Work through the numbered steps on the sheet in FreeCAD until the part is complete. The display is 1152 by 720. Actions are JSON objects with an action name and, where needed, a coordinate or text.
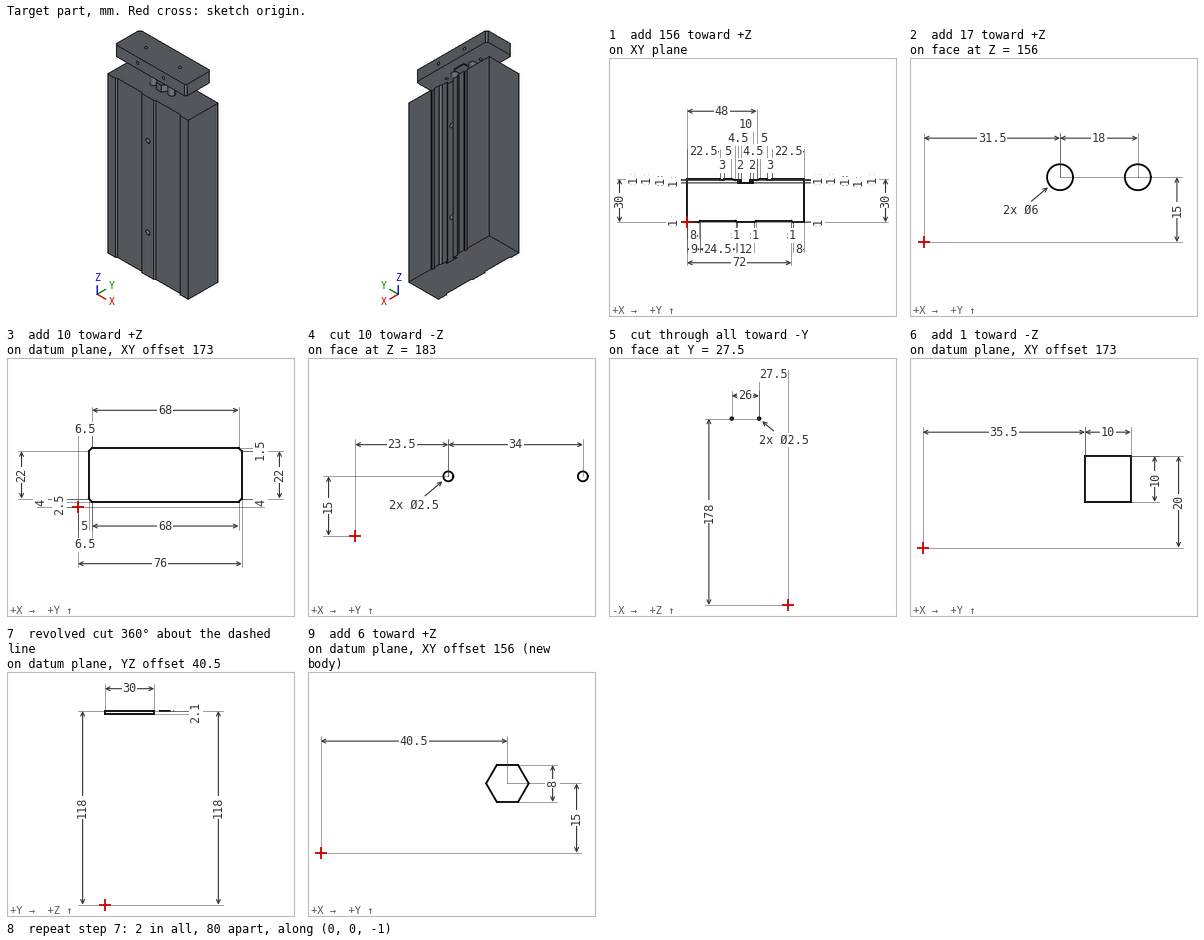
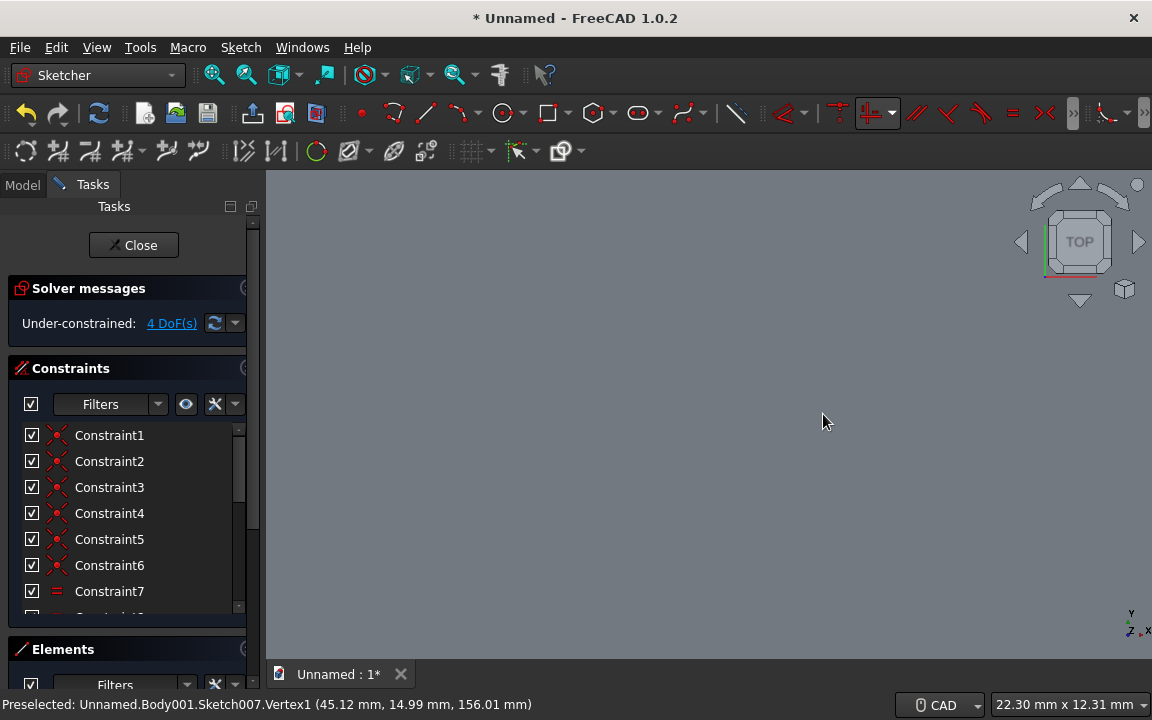
{"action": "left_click", "coordinate": [676, 256]}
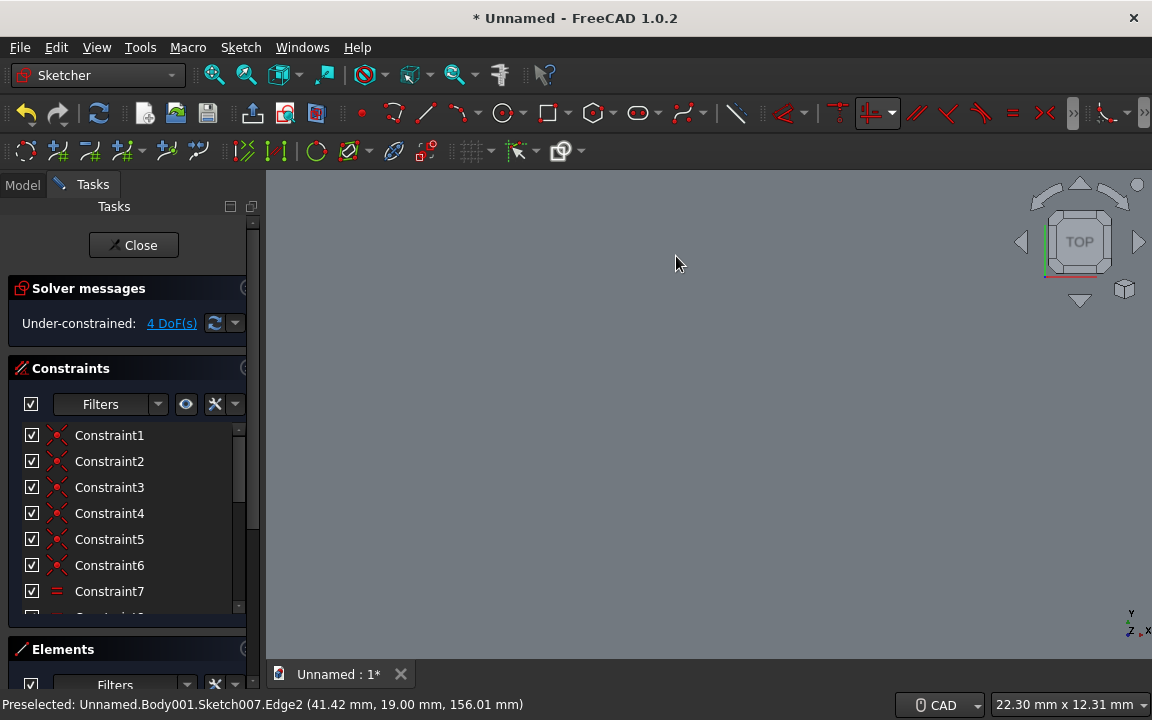
{"action": "key", "text": "h"}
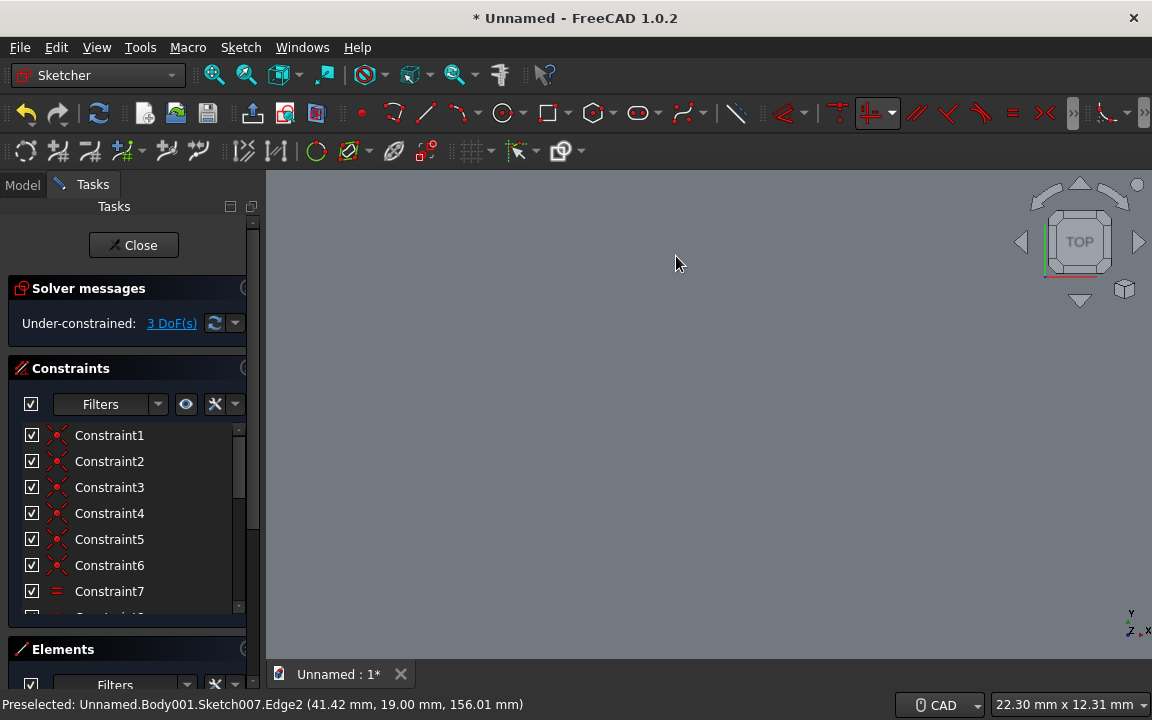
{"action": "left_click", "coordinate": [784, 114]}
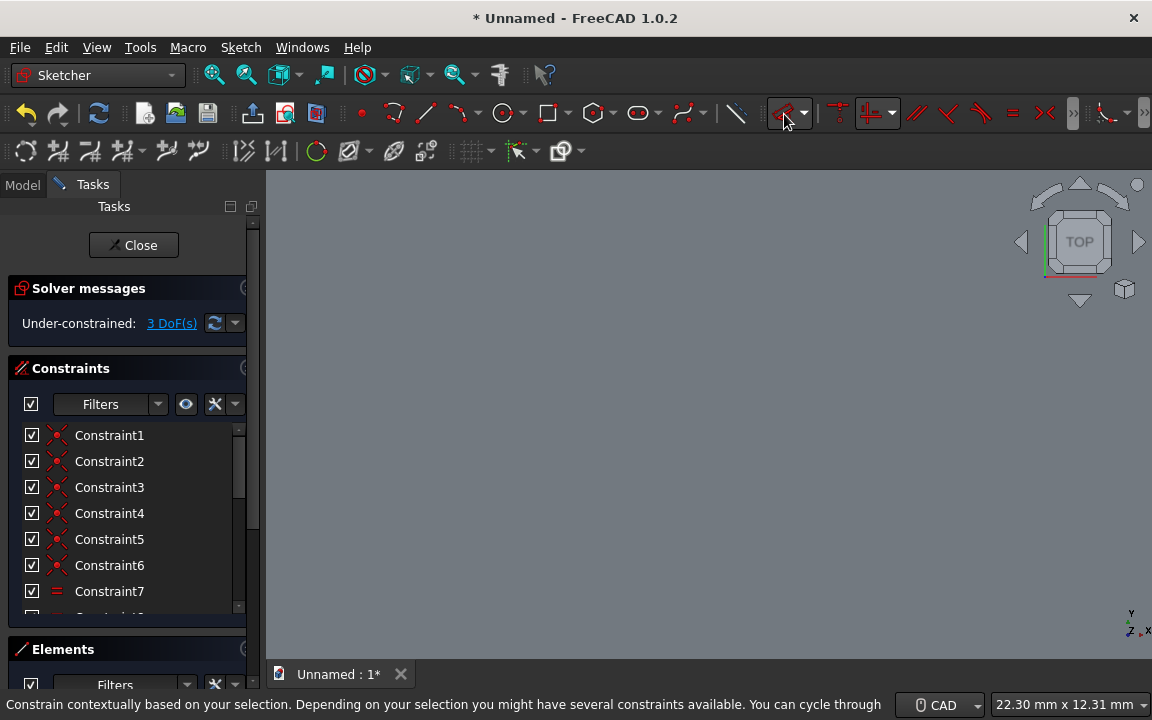
{"action": "left_click", "coordinate": [547, 574]}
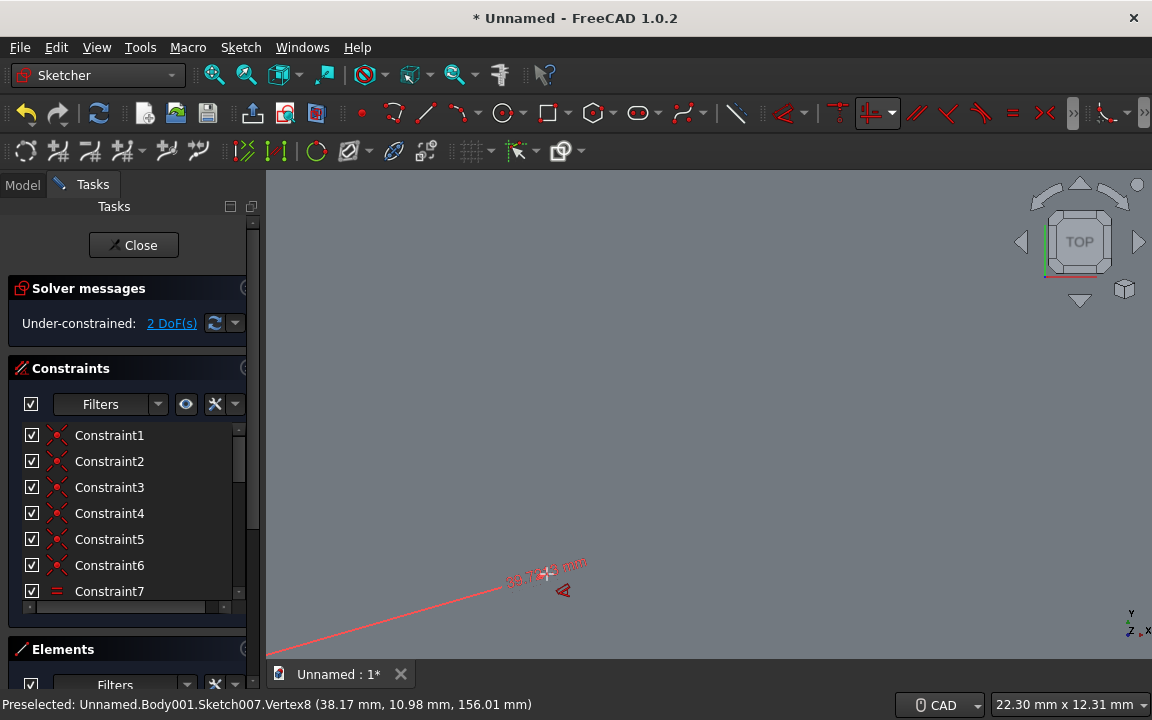
{"action": "left_click", "coordinate": [731, 256]}
{"action": "left_click", "coordinate": [513, 415]}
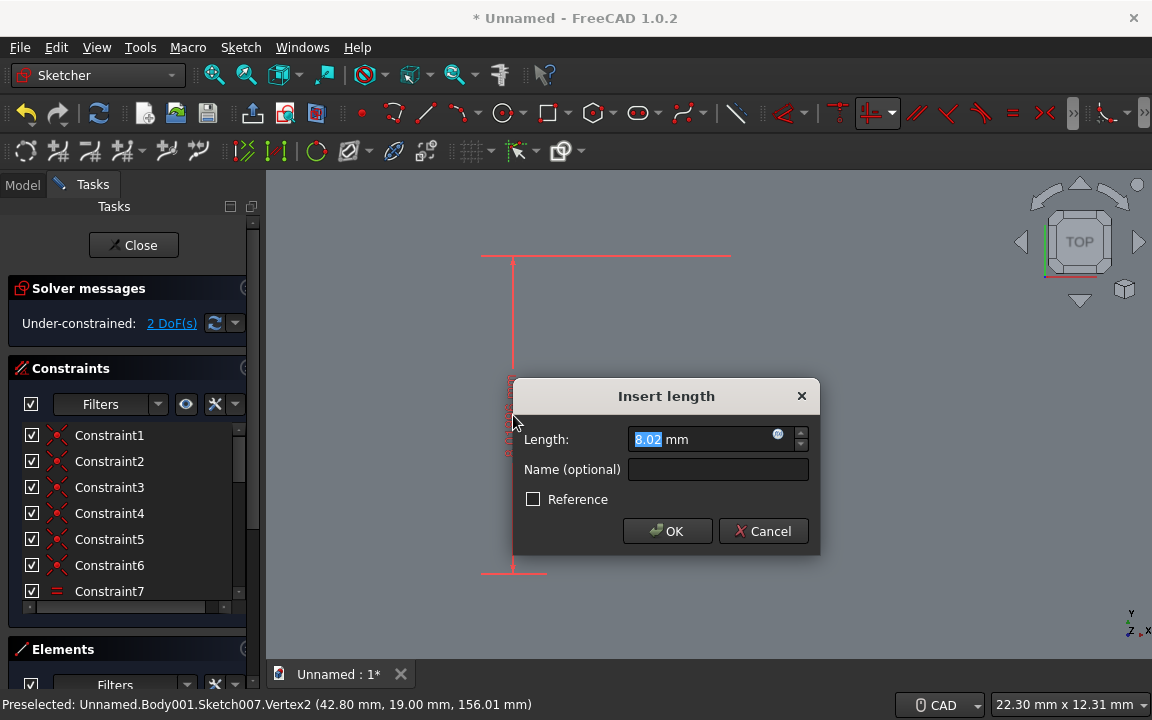
{"action": "type", "text": "8"}
{"action": "key", "text": "Return"}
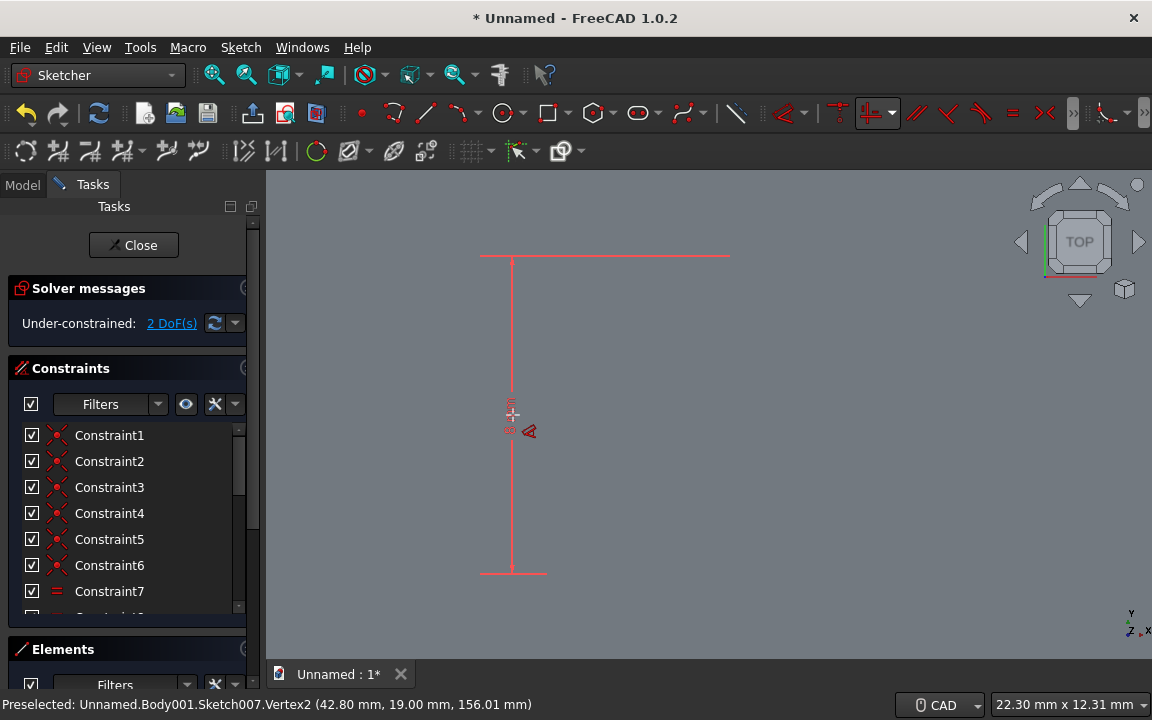
{"action": "left_click", "coordinate": [639, 415]}
{"action": "left_click", "coordinate": [673, 523]}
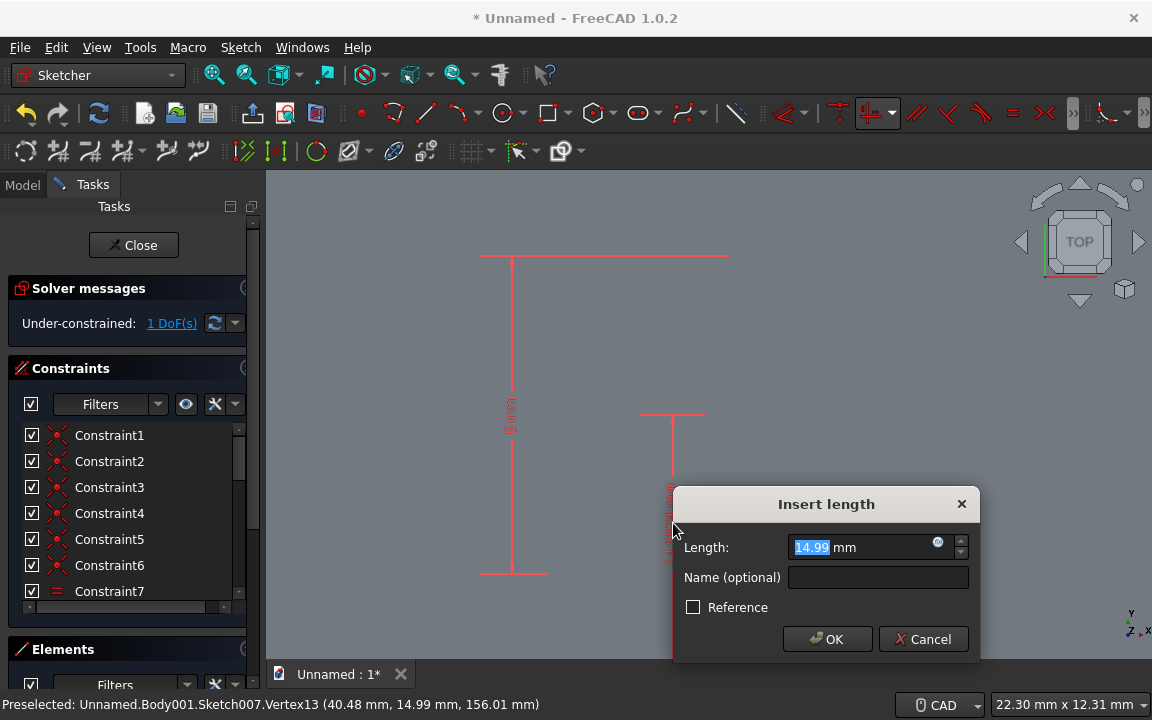
{"action": "type", "text": "15"}
{"action": "key", "text": "Return"}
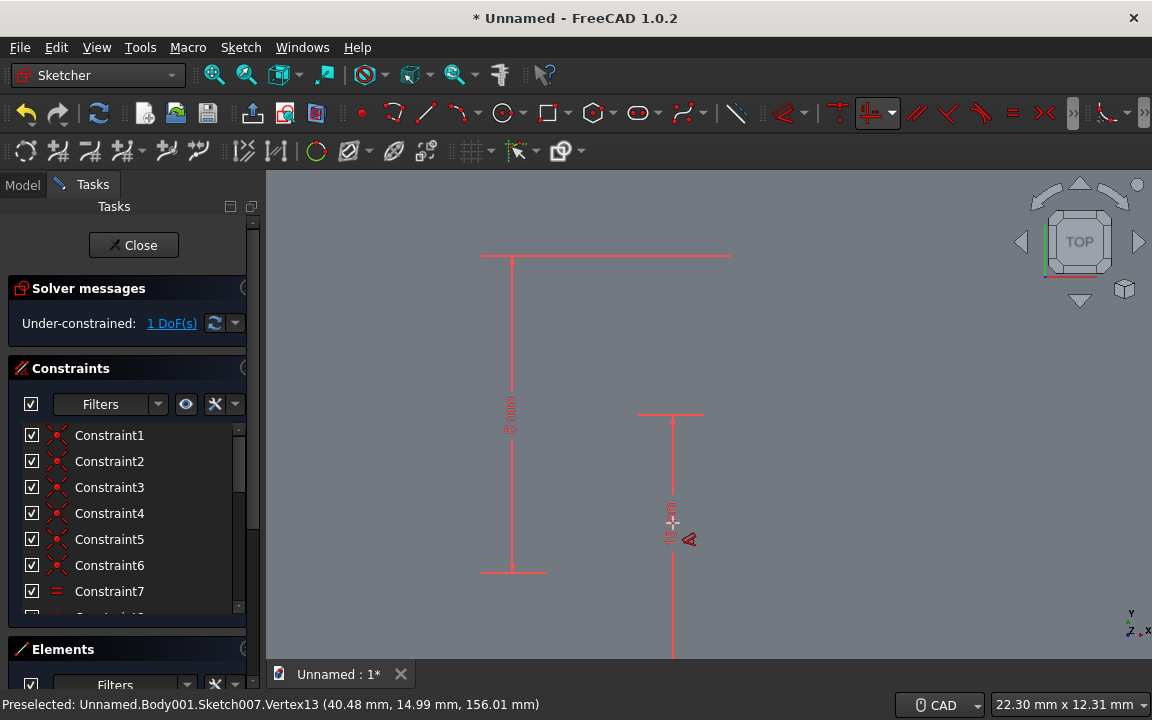
{"action": "left_click", "coordinate": [639, 414]}
{"action": "left_click", "coordinate": [387, 380]}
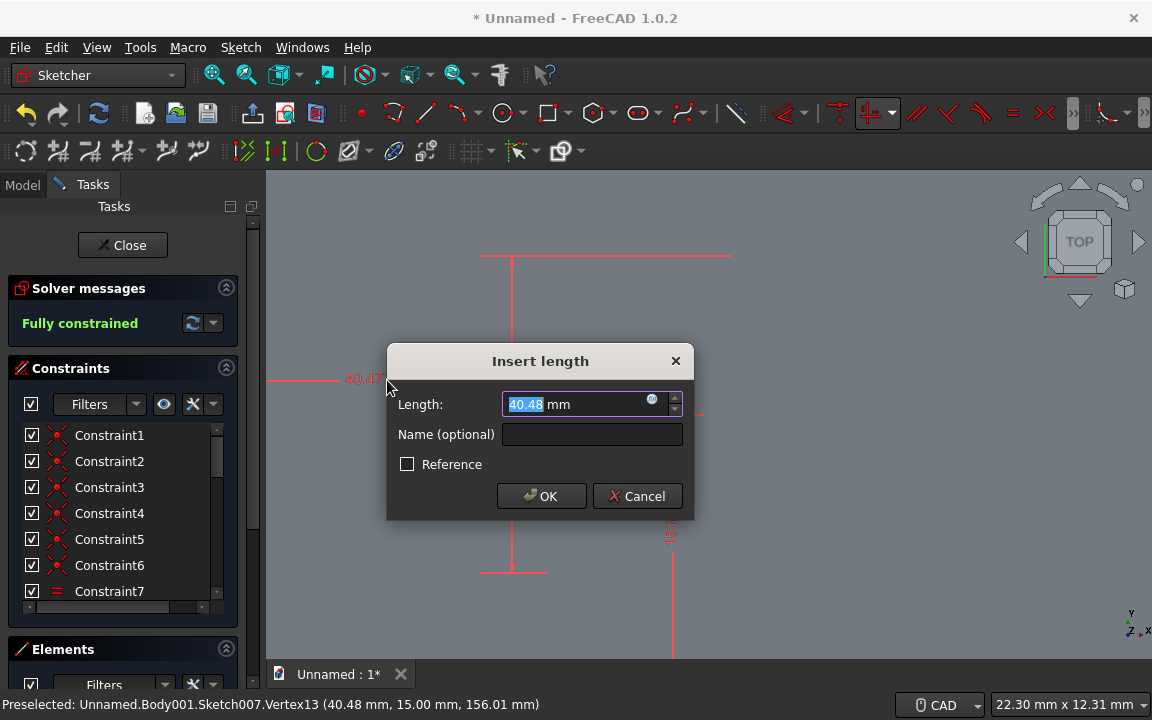
{"action": "type", "text": "40.5"}
{"action": "key", "text": "Return"}
{"action": "key", "text": "Escape"}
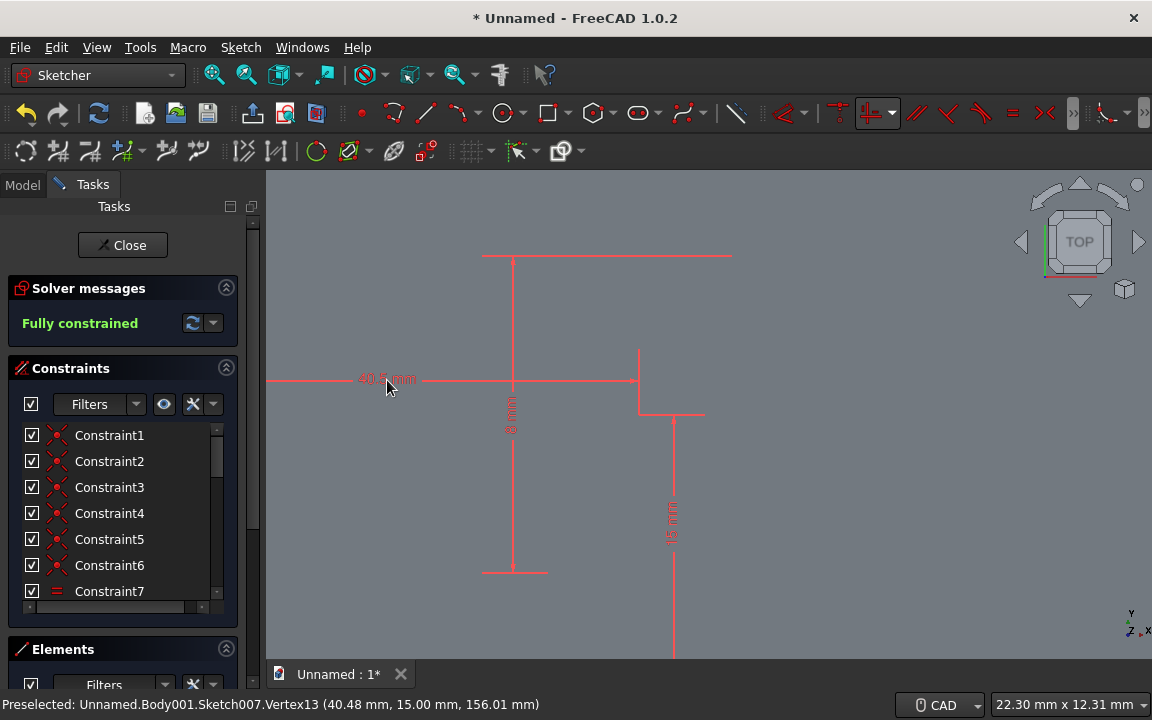
{"action": "left_click", "coordinate": [123, 245]}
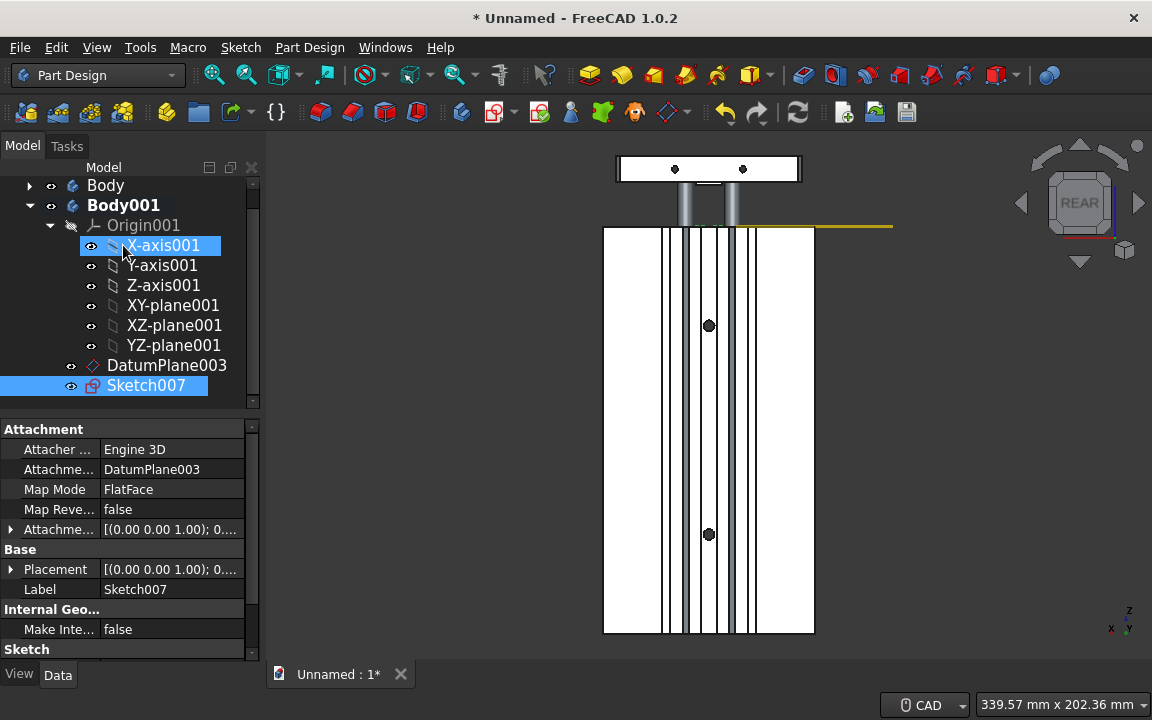
{"action": "left_click", "coordinate": [590, 76]}